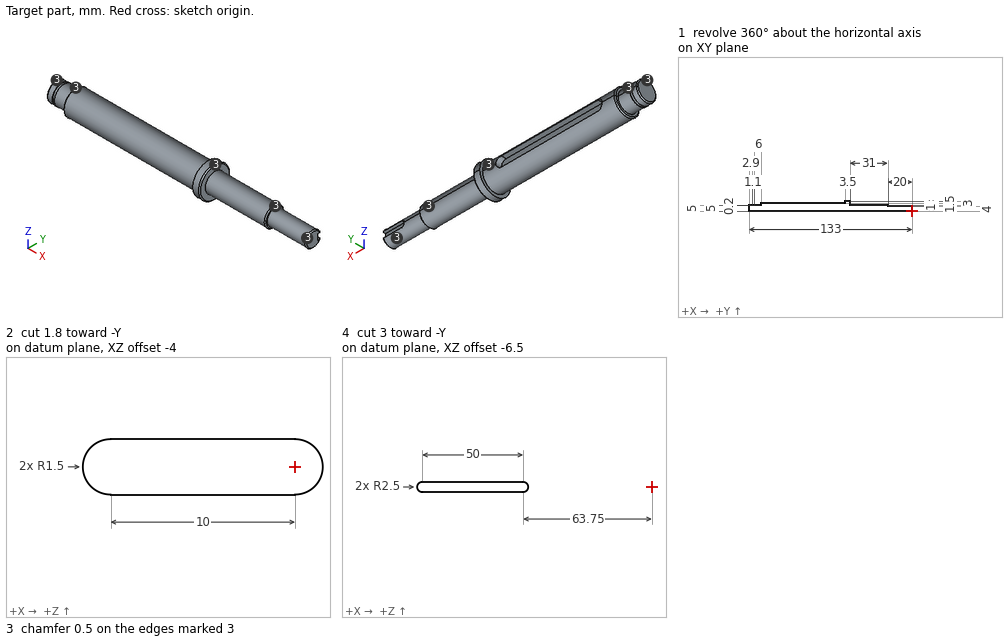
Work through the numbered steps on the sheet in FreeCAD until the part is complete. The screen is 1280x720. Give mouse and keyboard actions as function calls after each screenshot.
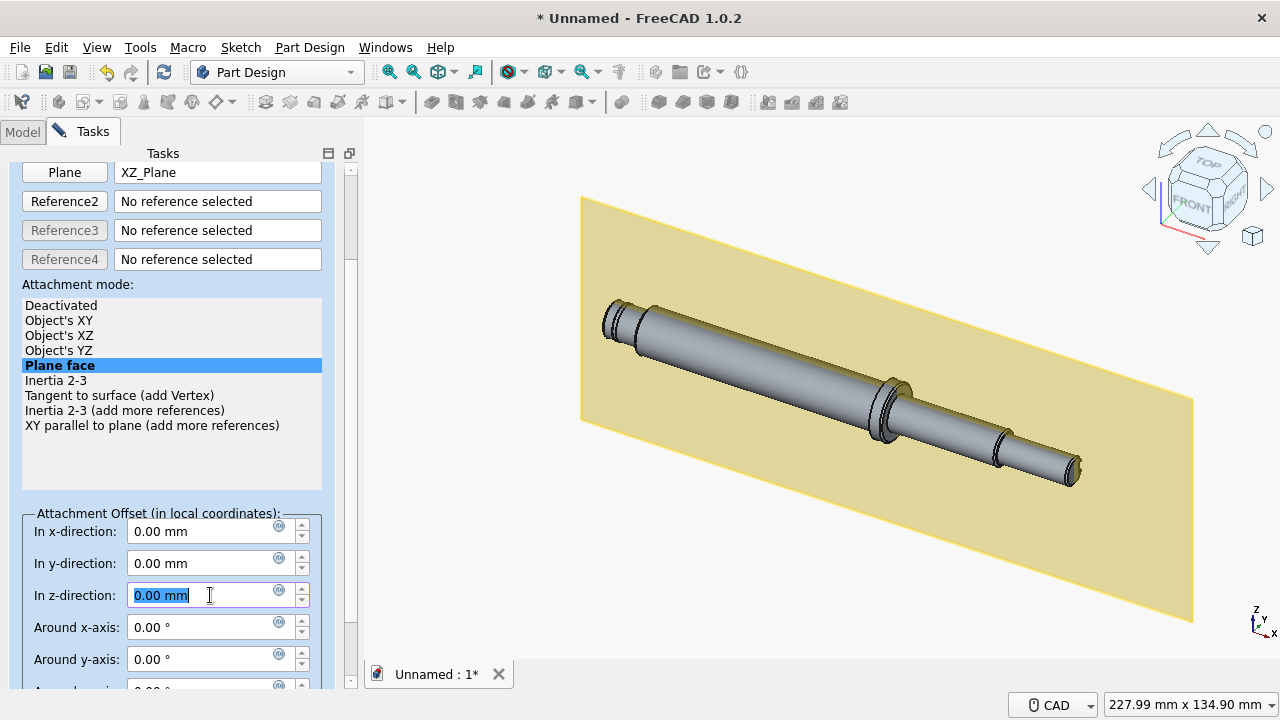
text(-6.5)
key(Tab)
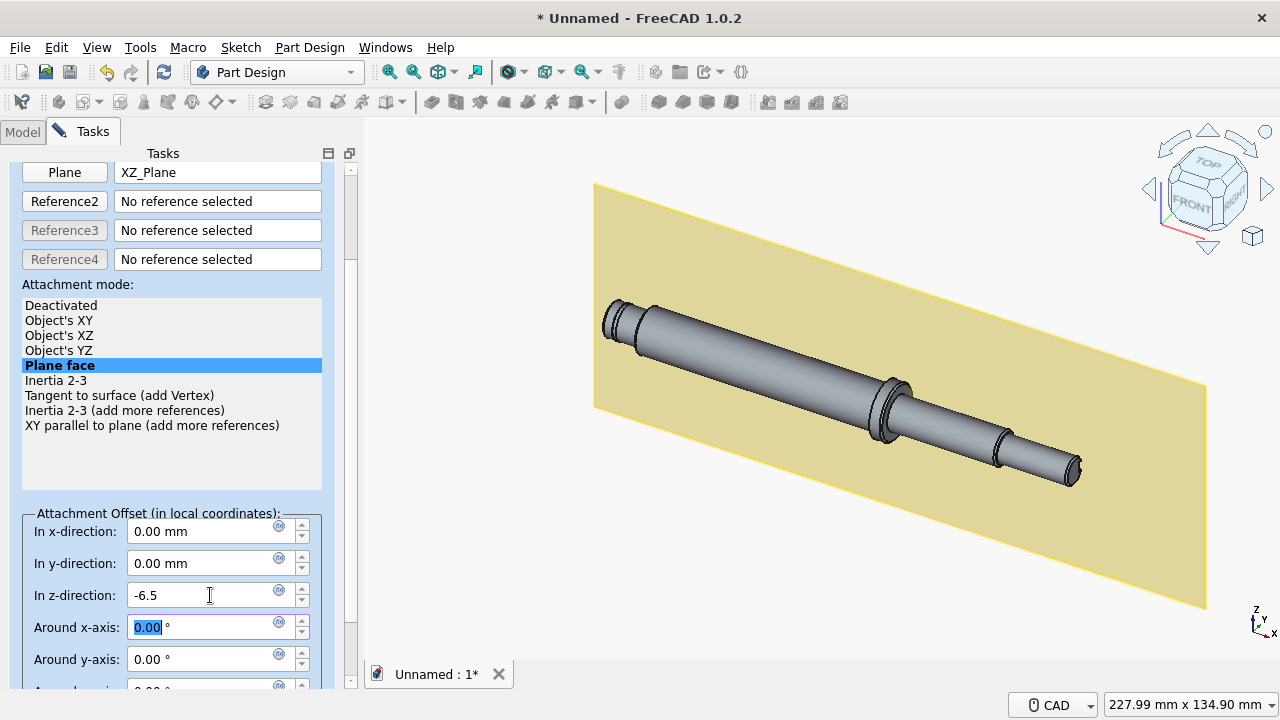
scroll(351, 426, up, 3)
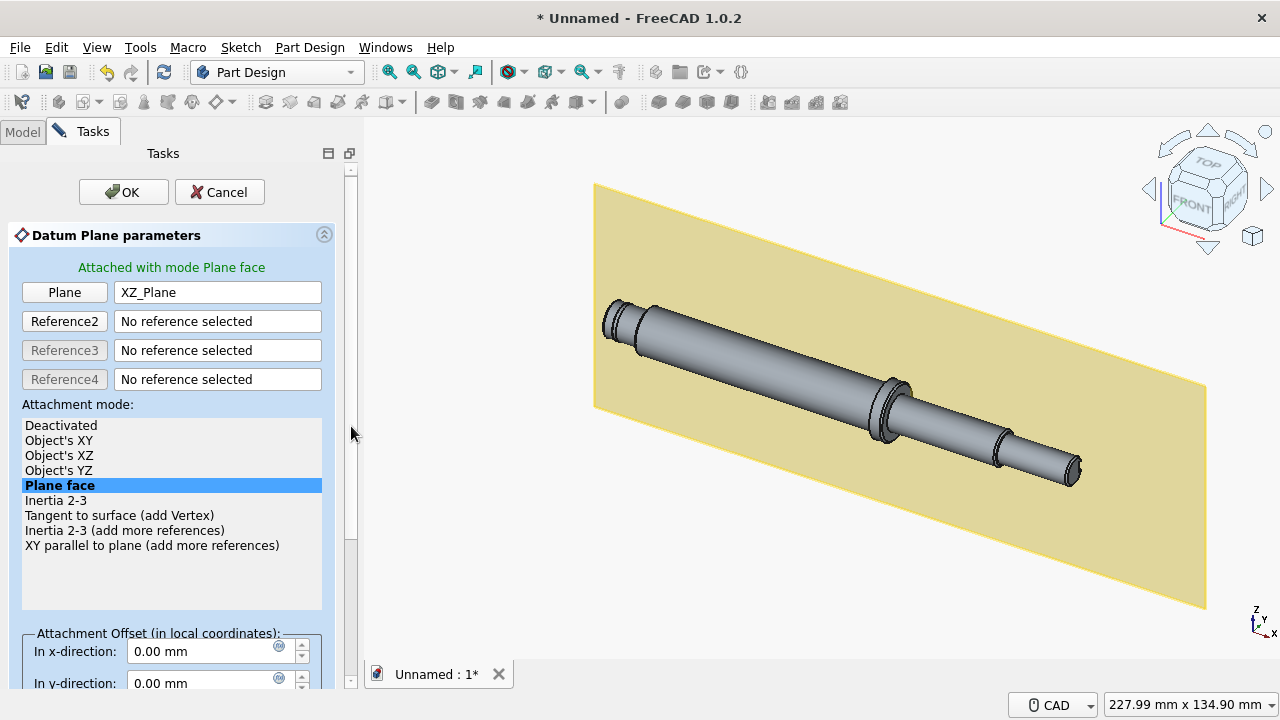
click(124, 192)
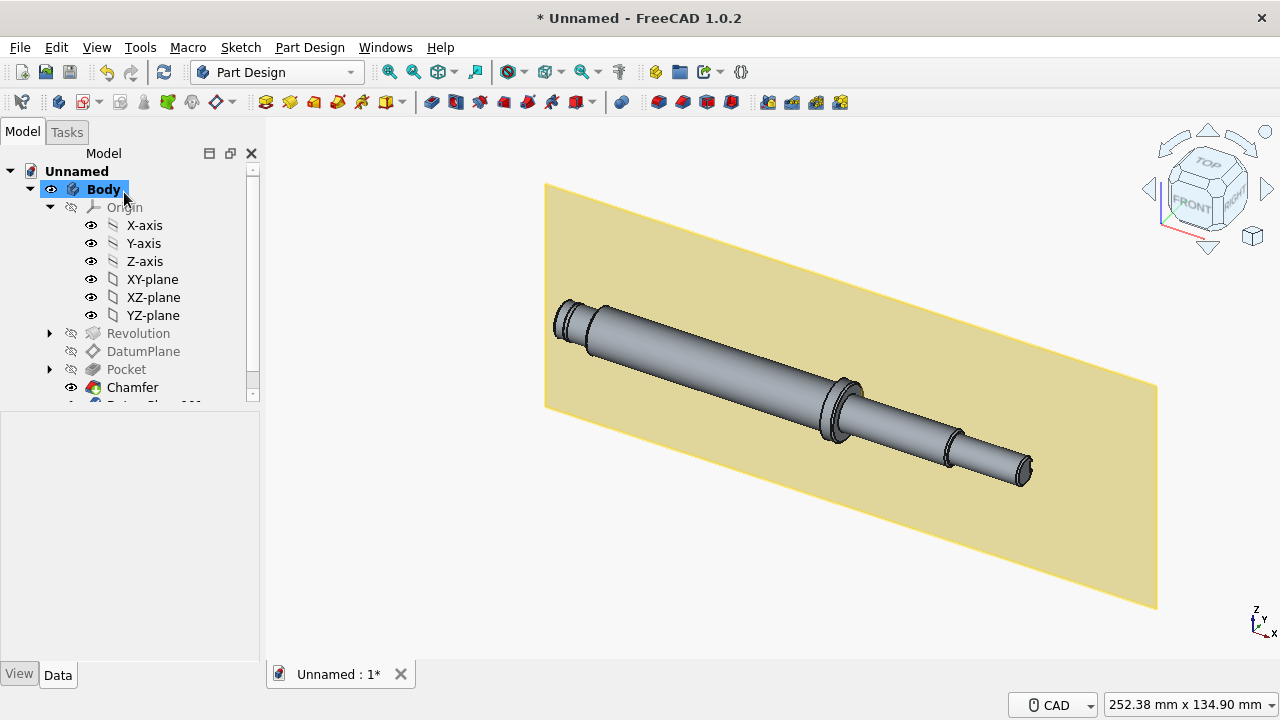
scroll(100, 275, down, 3)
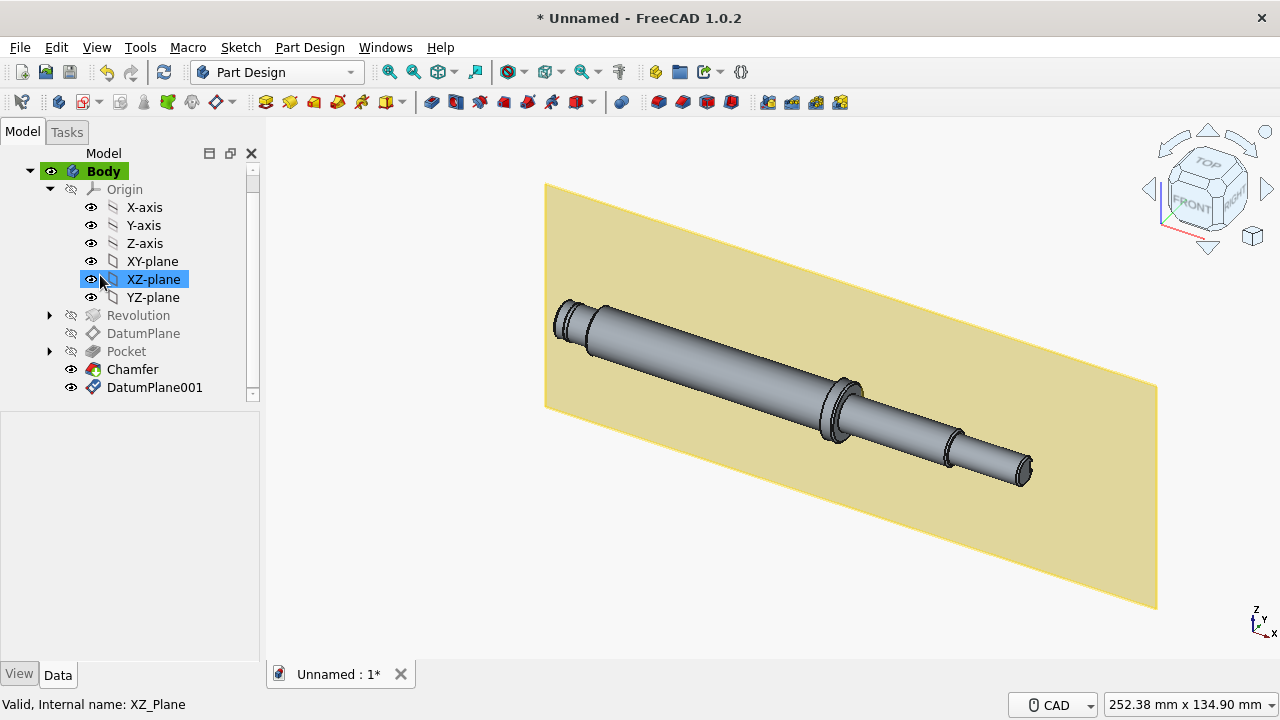
click(116, 387)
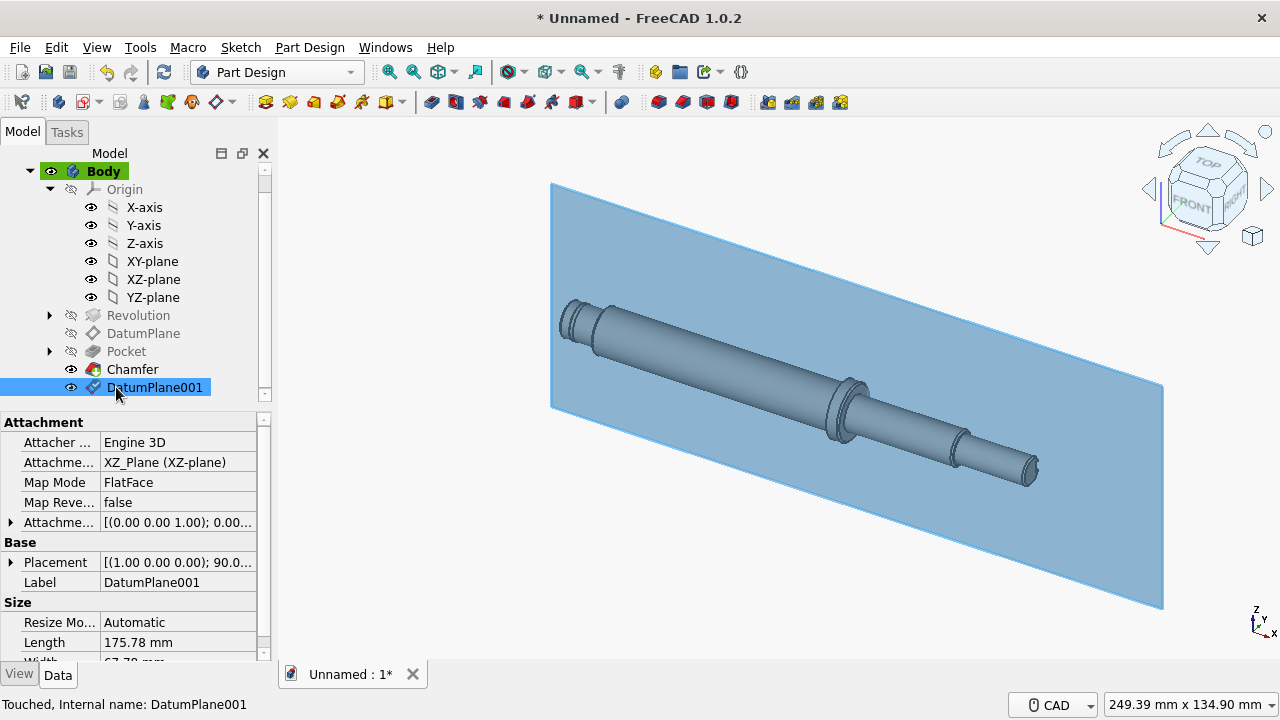
click(84, 102)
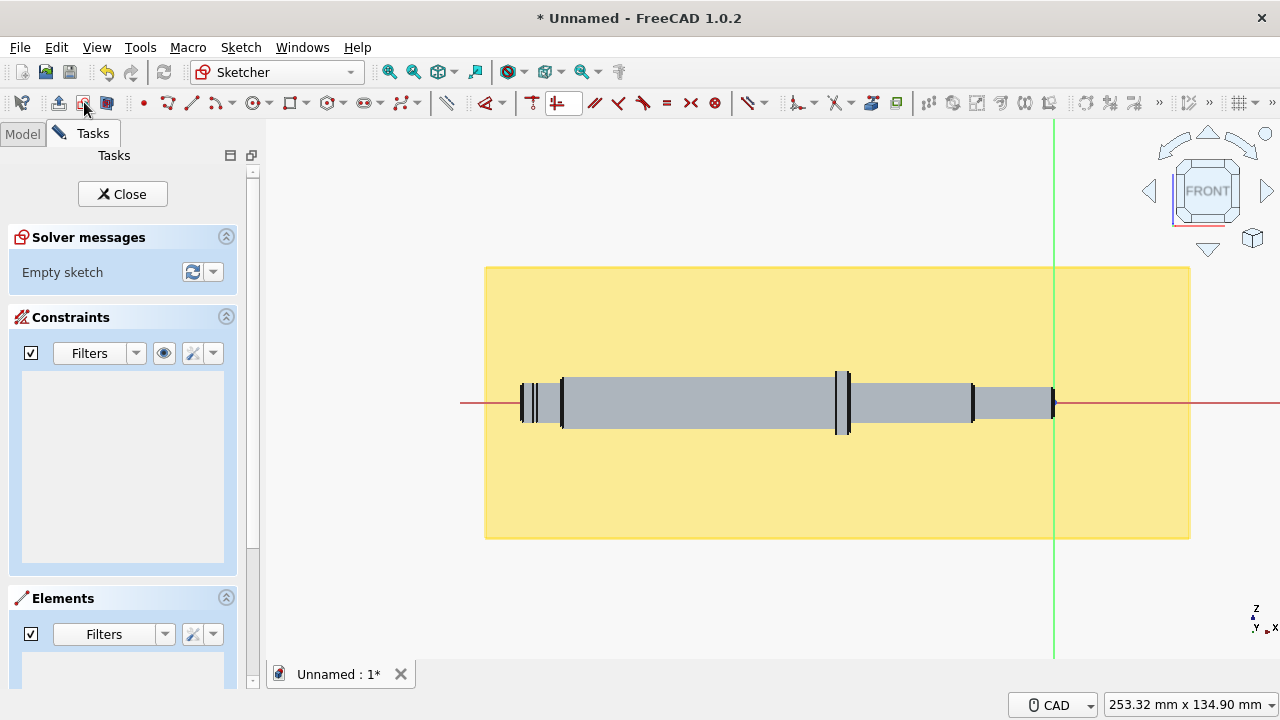
key(q)
key(s)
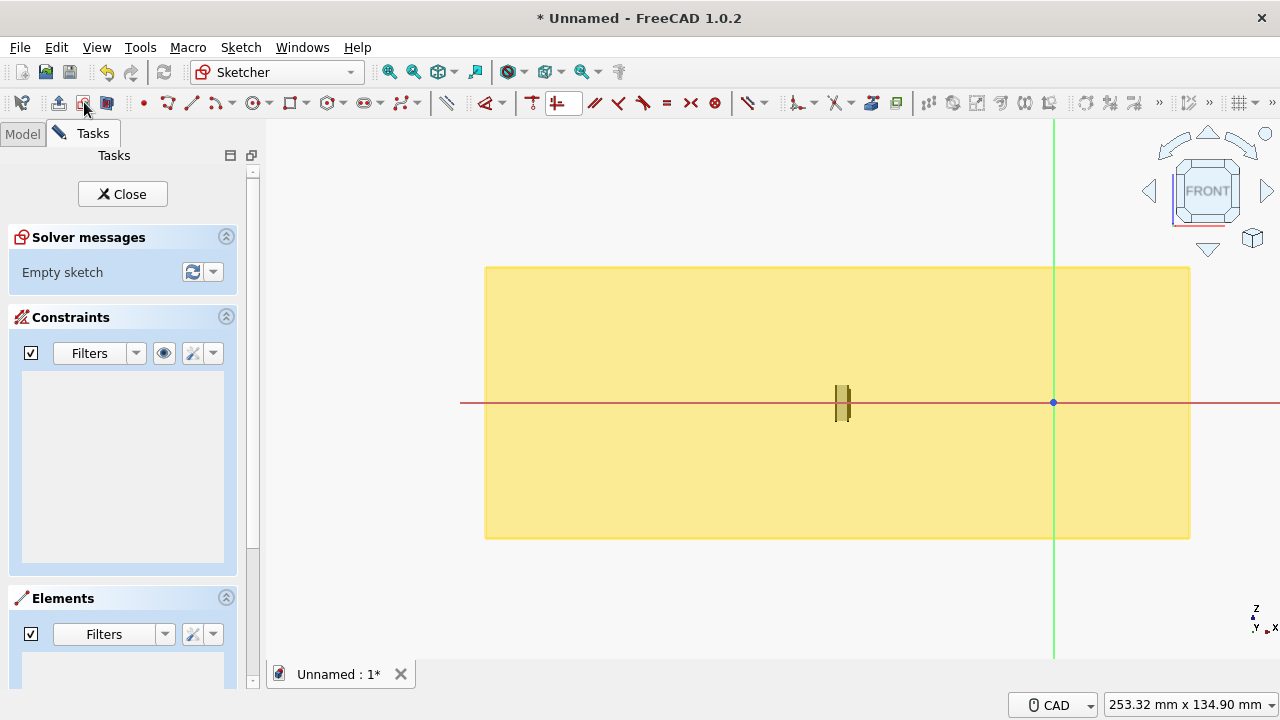
click(364, 104)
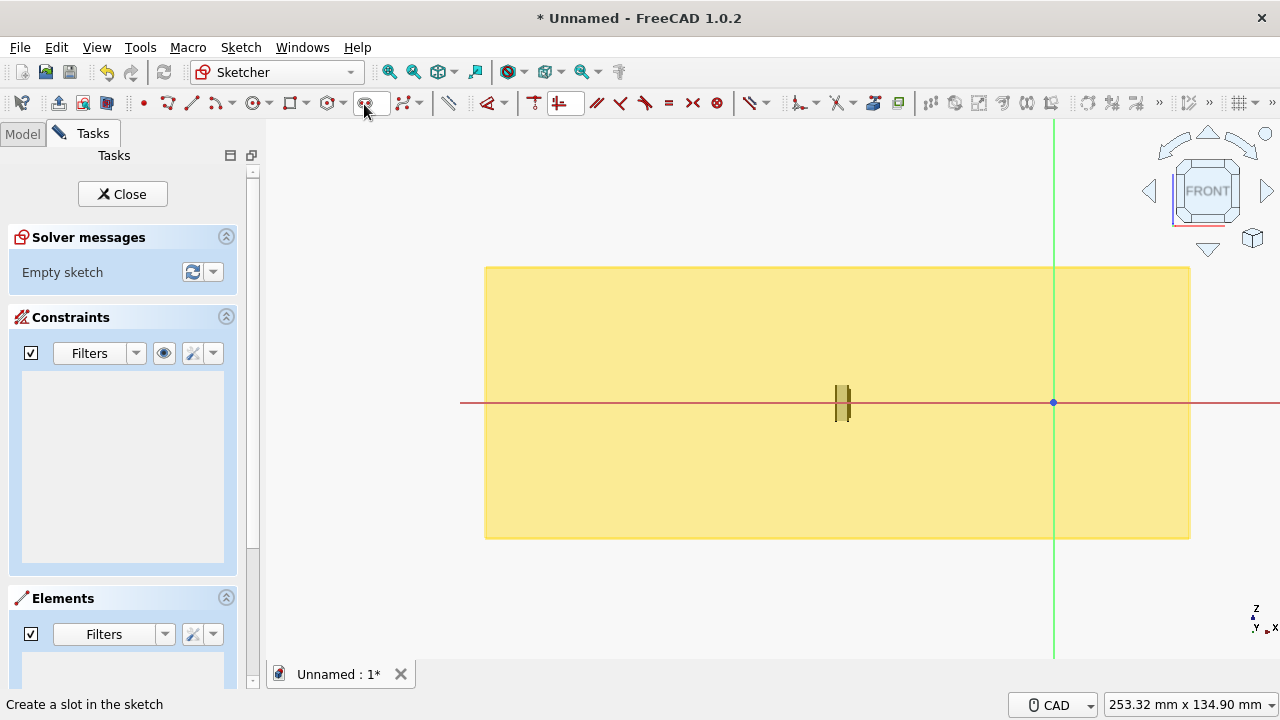
scroll(598, 403, up, 5)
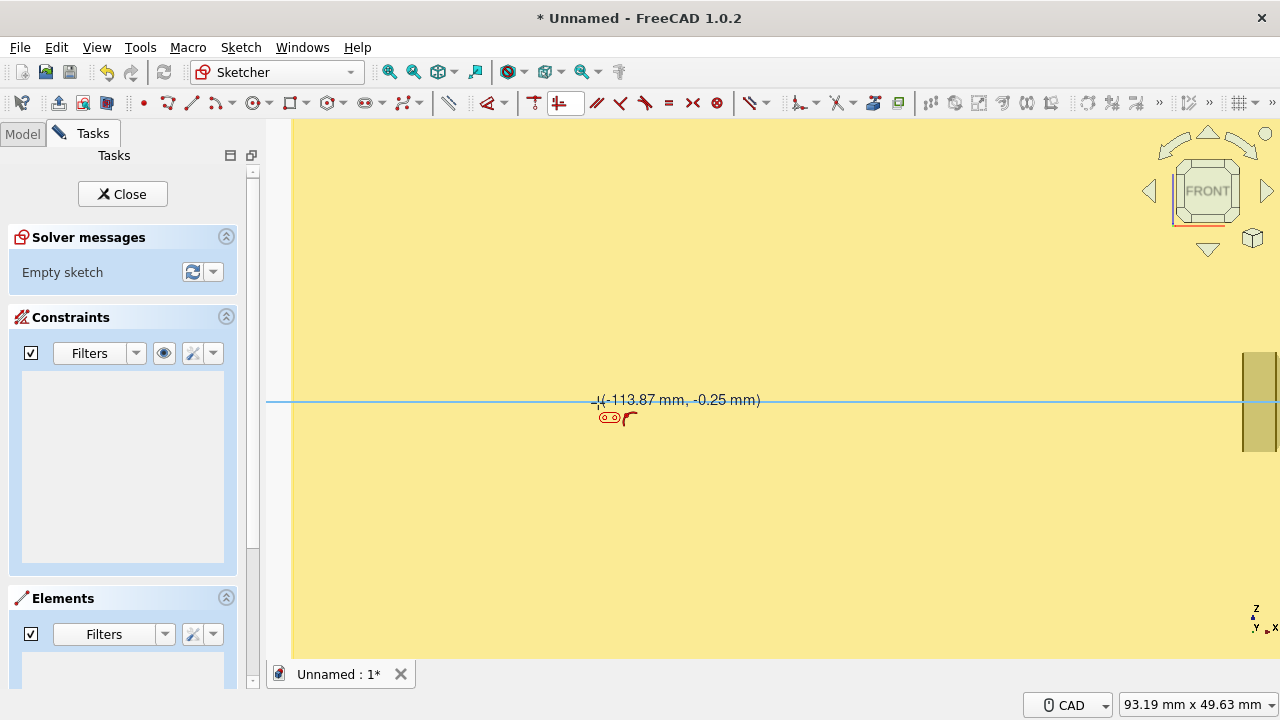
click(599, 402)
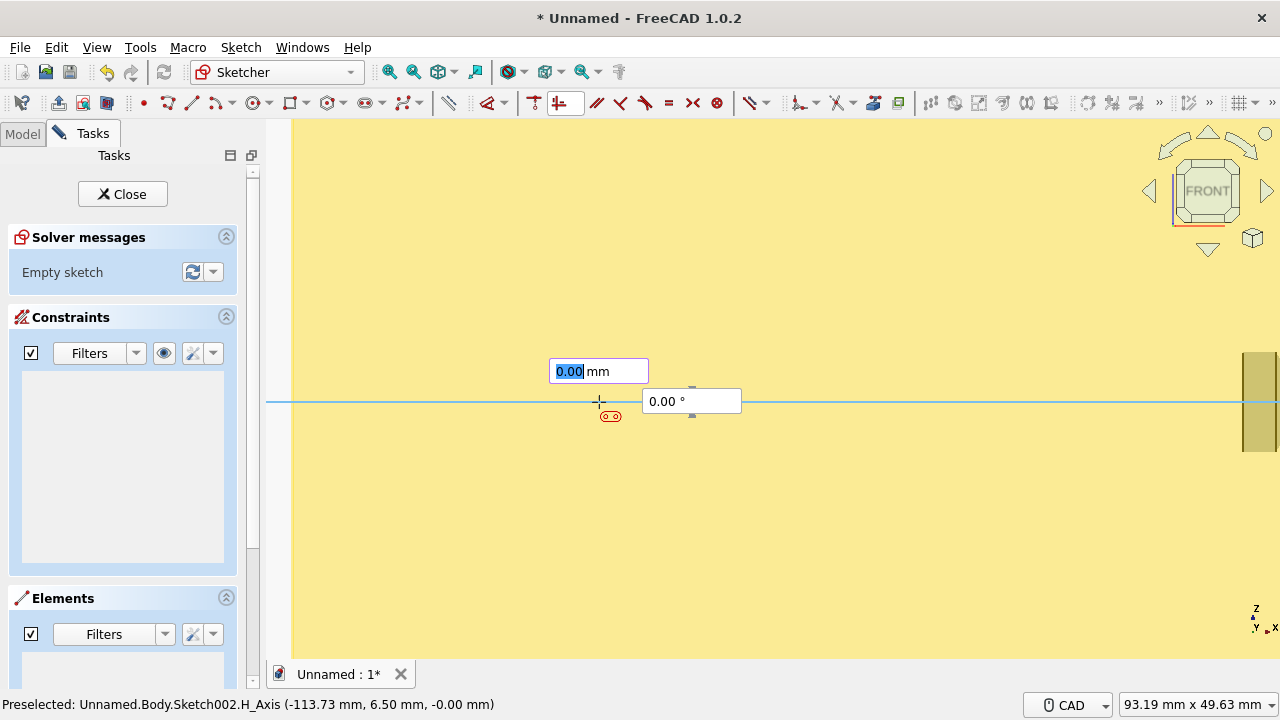
scroll(297, 378, down, 4)